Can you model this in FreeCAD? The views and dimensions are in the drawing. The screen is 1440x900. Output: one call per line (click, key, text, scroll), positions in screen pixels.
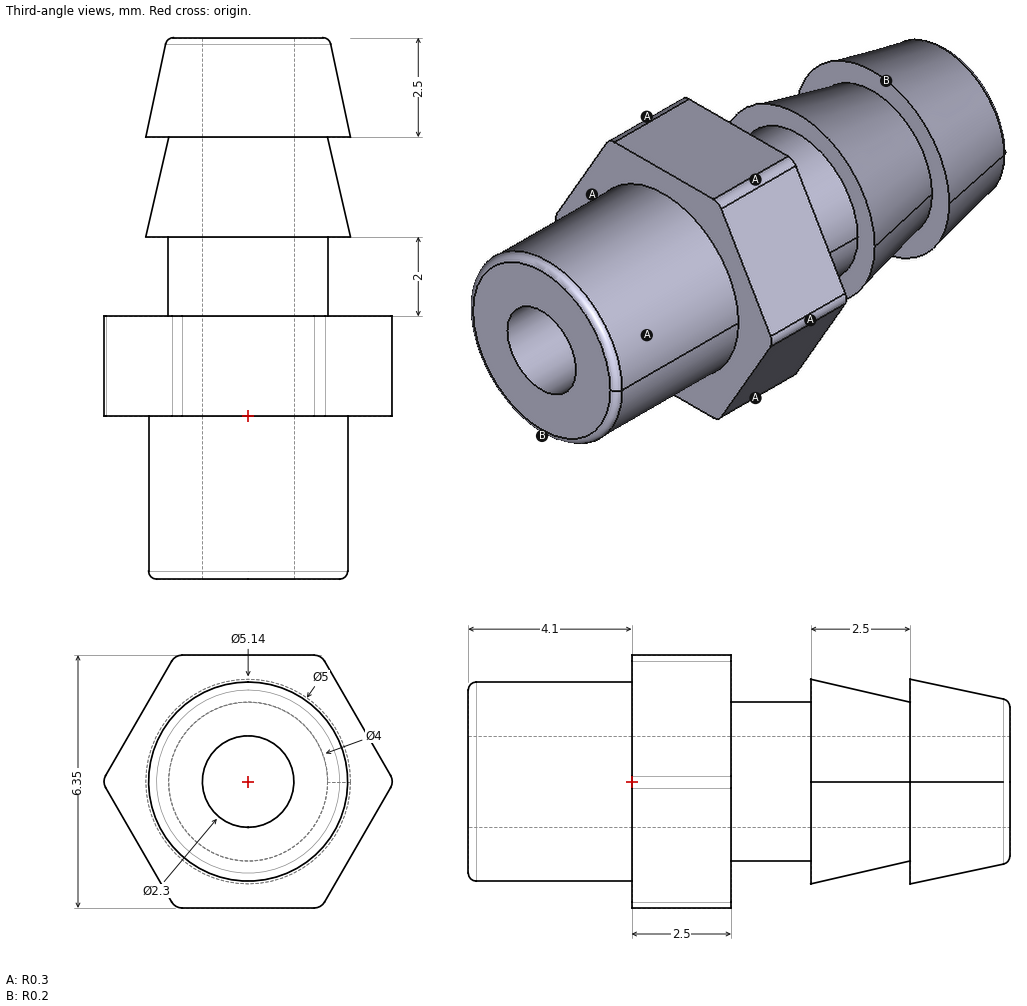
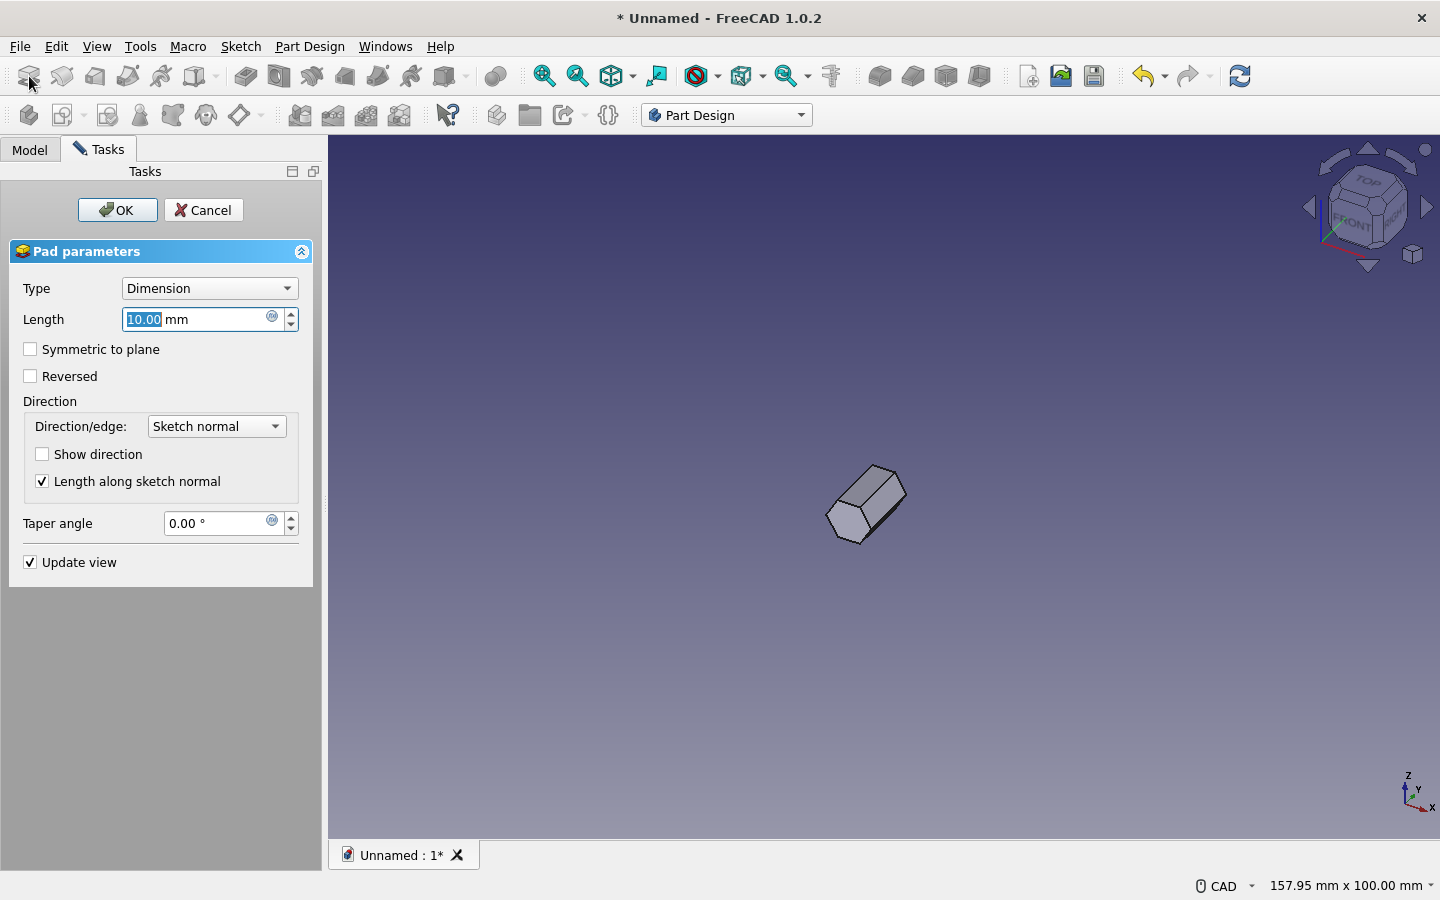
text(2.5)
key(Tab)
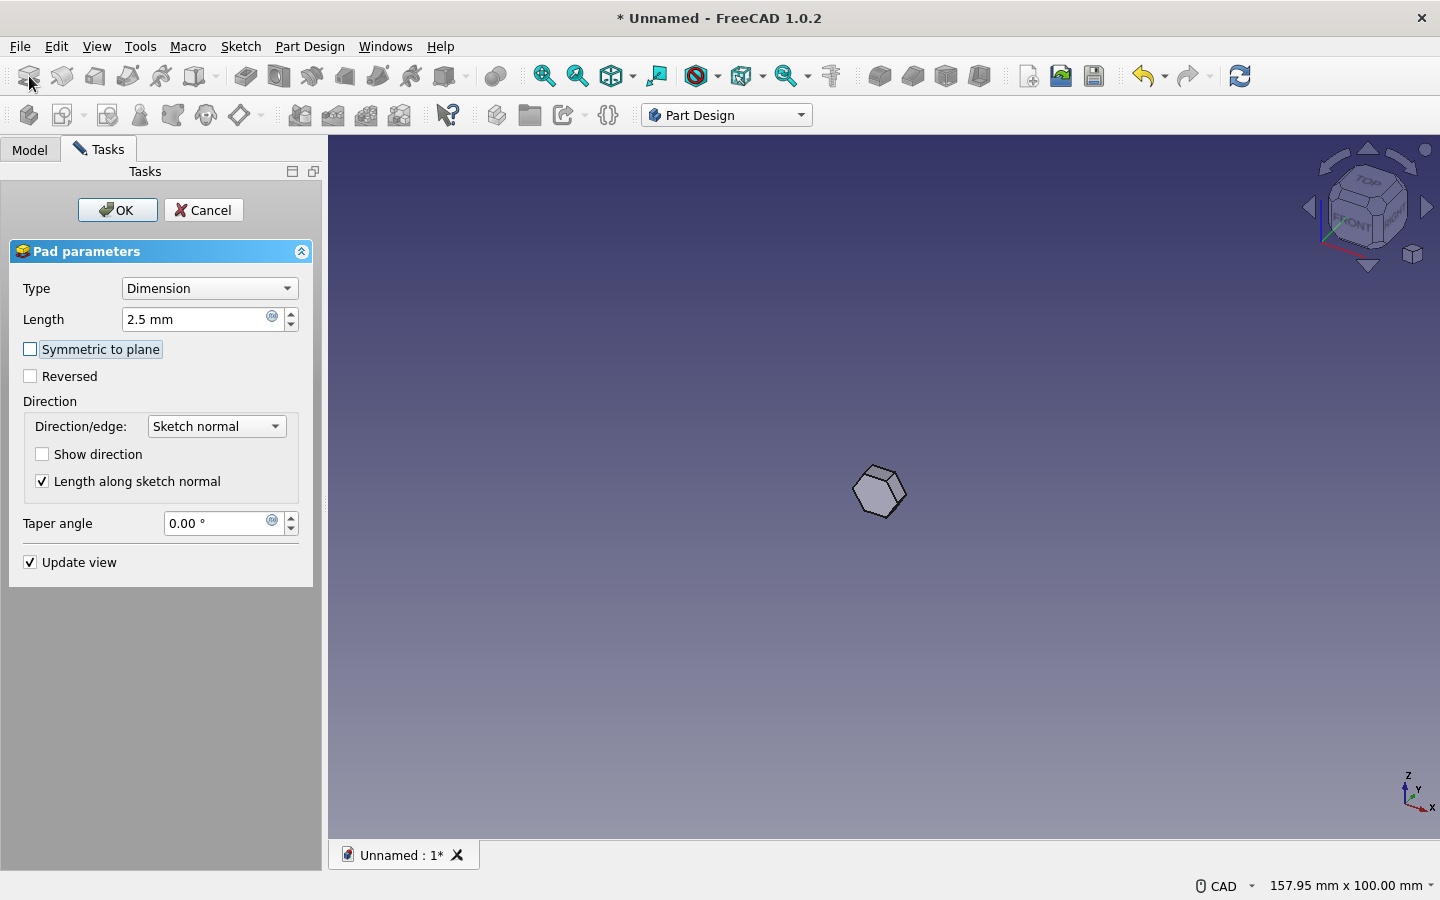
click(31, 376)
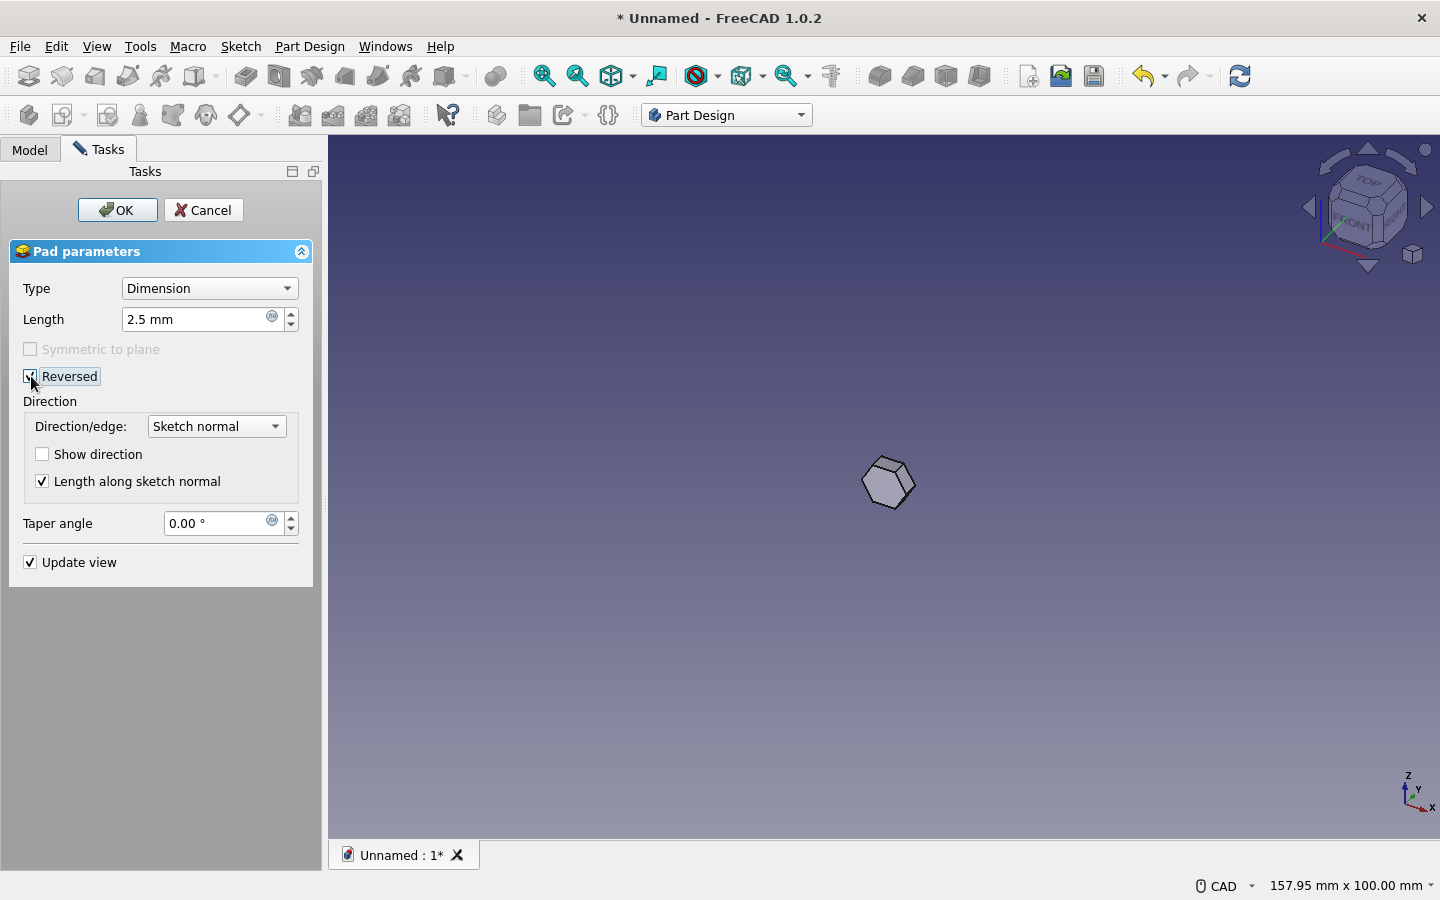
click(118, 210)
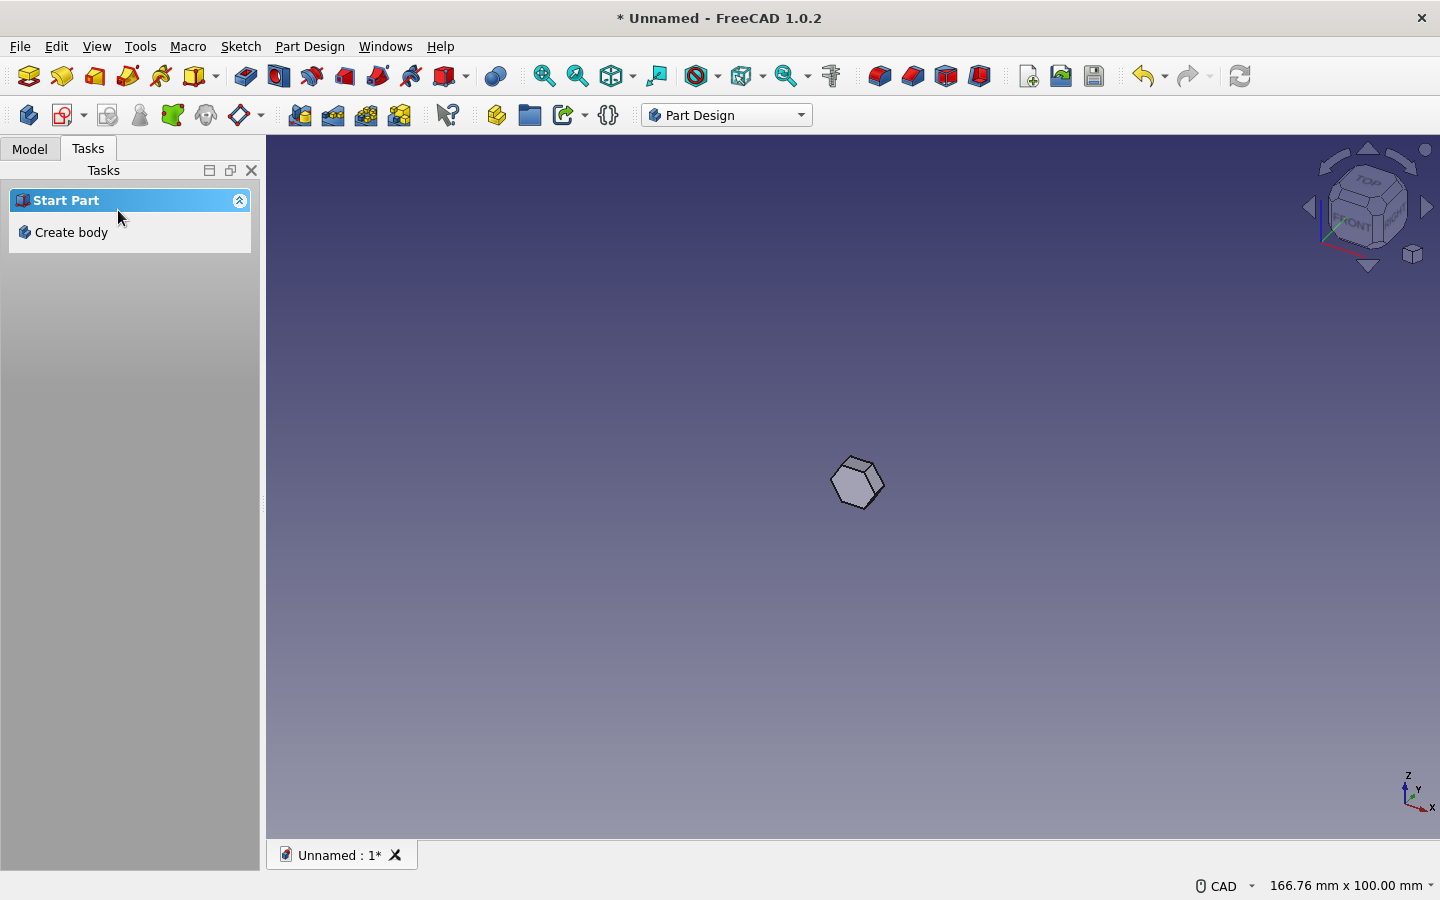
click(545, 76)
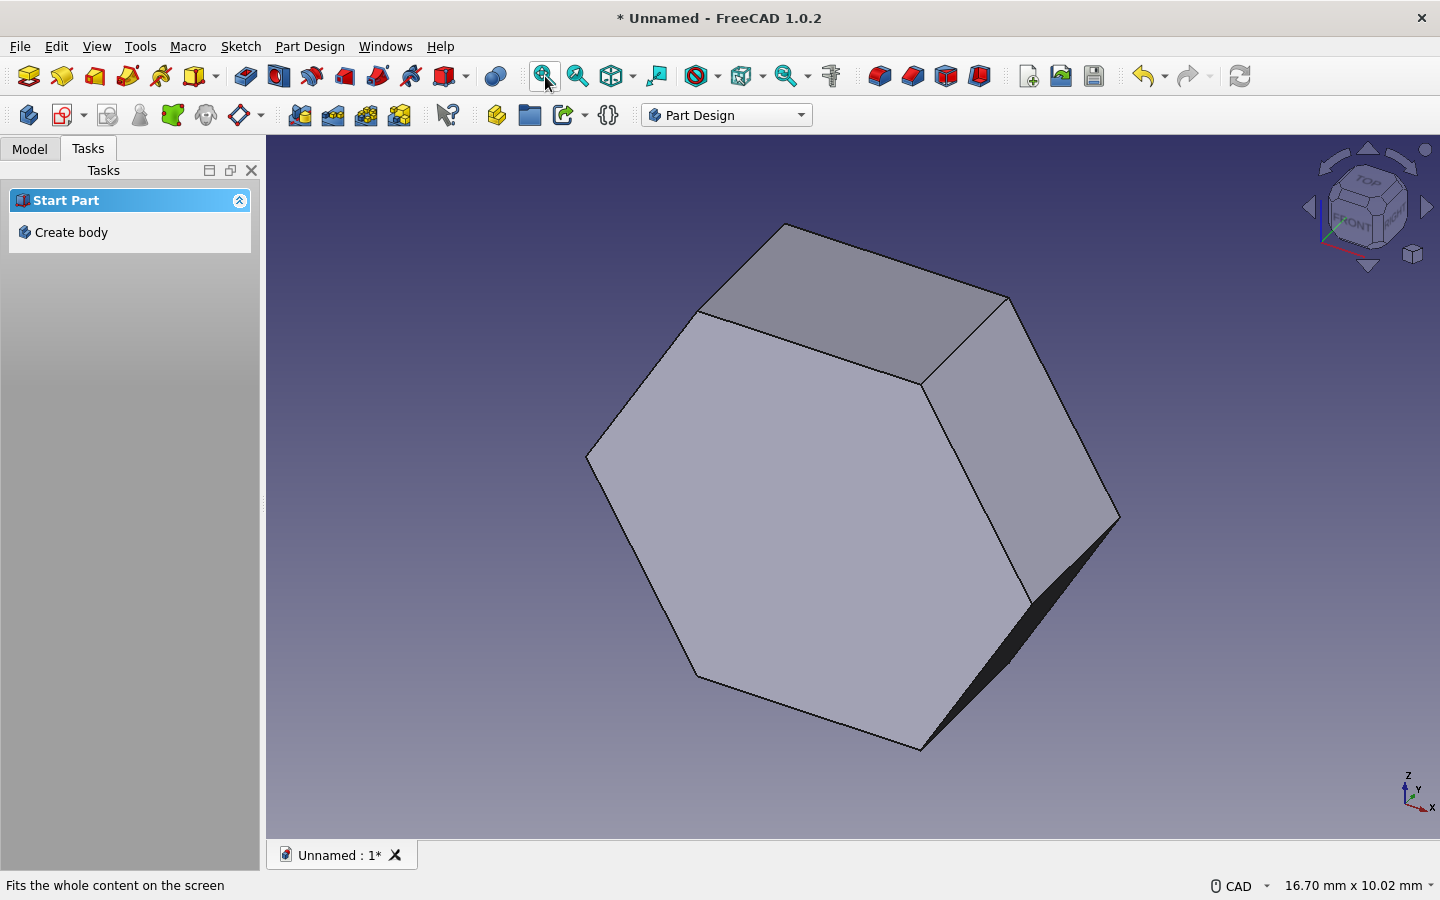
key(4)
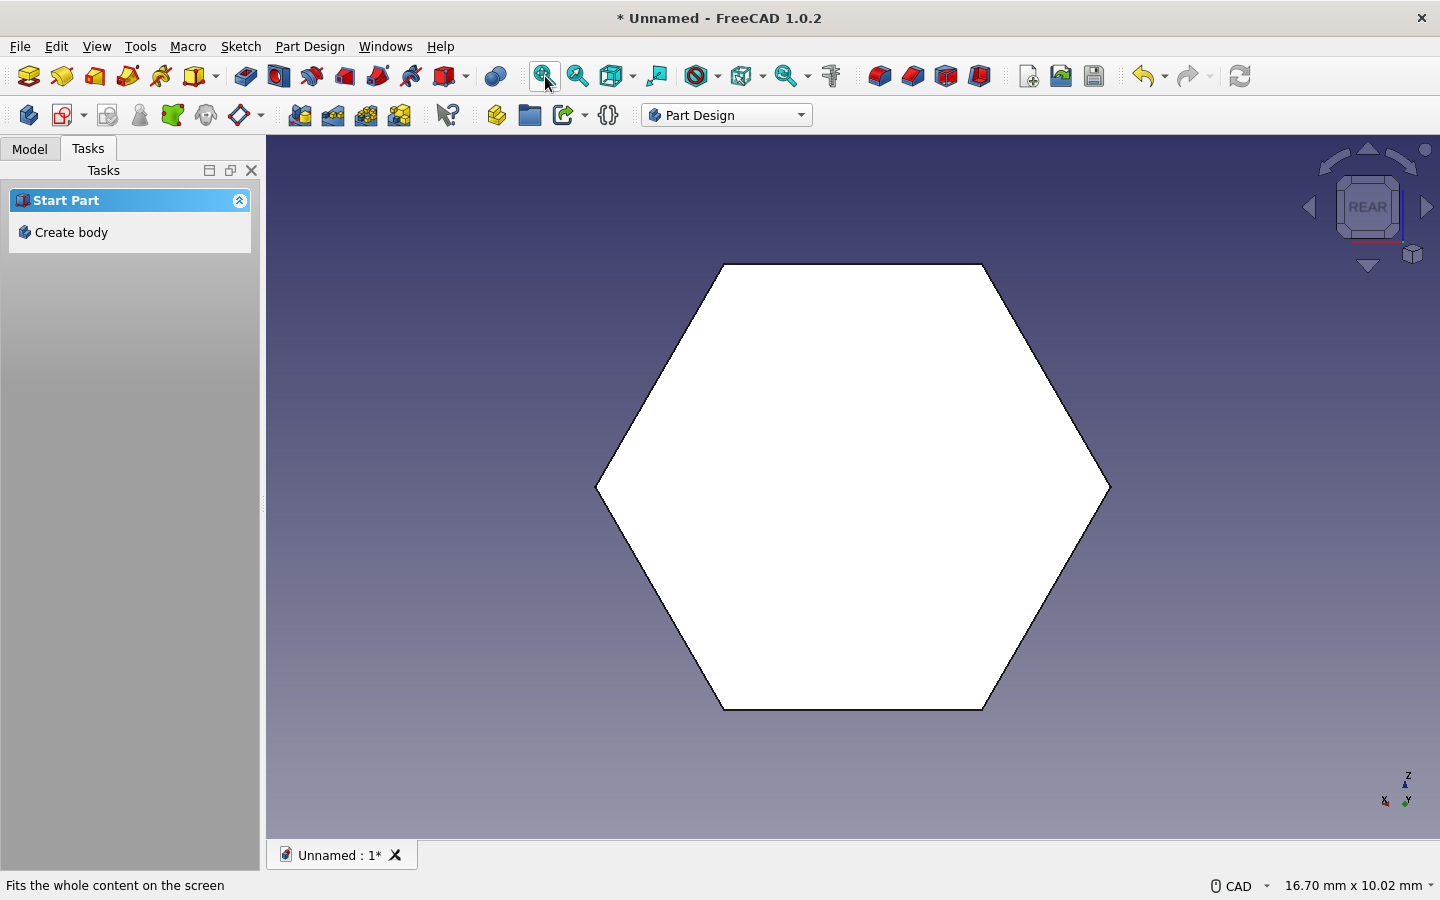
click(853, 486)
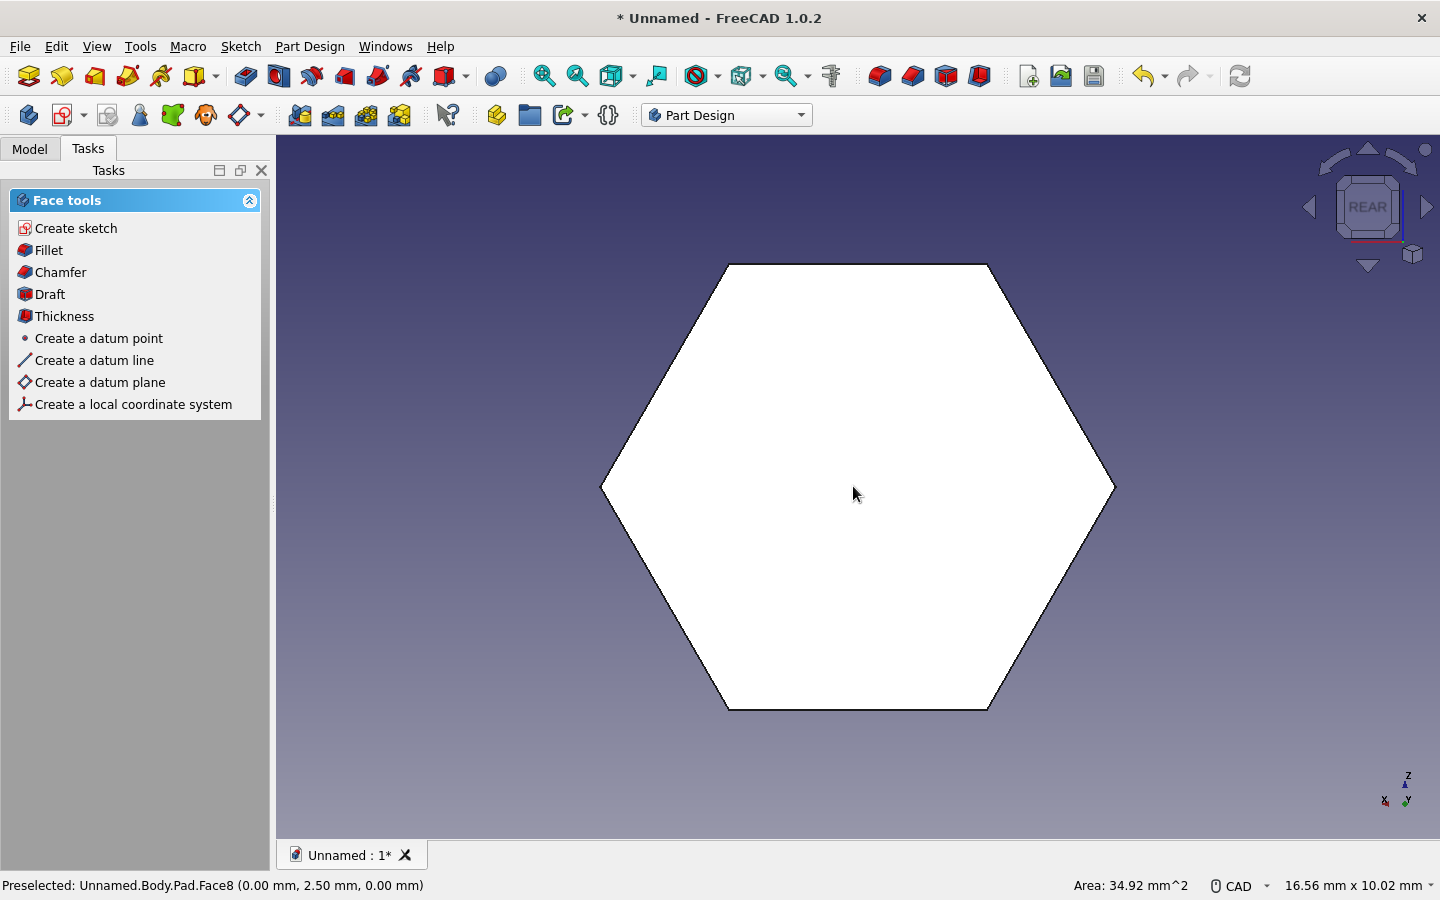
click(62, 116)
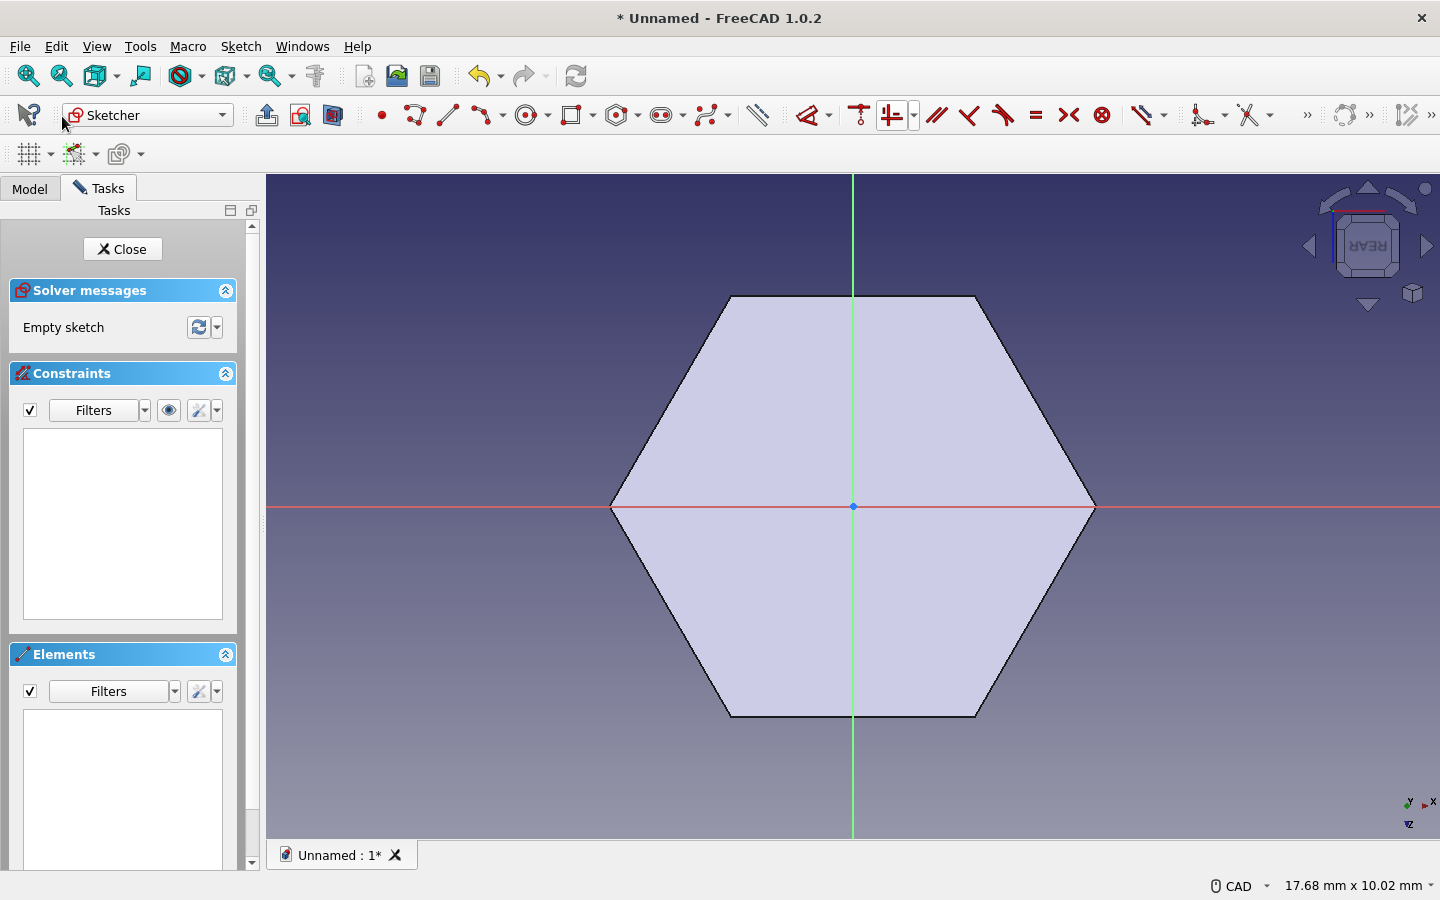
scroll(992, 506, up, 2)